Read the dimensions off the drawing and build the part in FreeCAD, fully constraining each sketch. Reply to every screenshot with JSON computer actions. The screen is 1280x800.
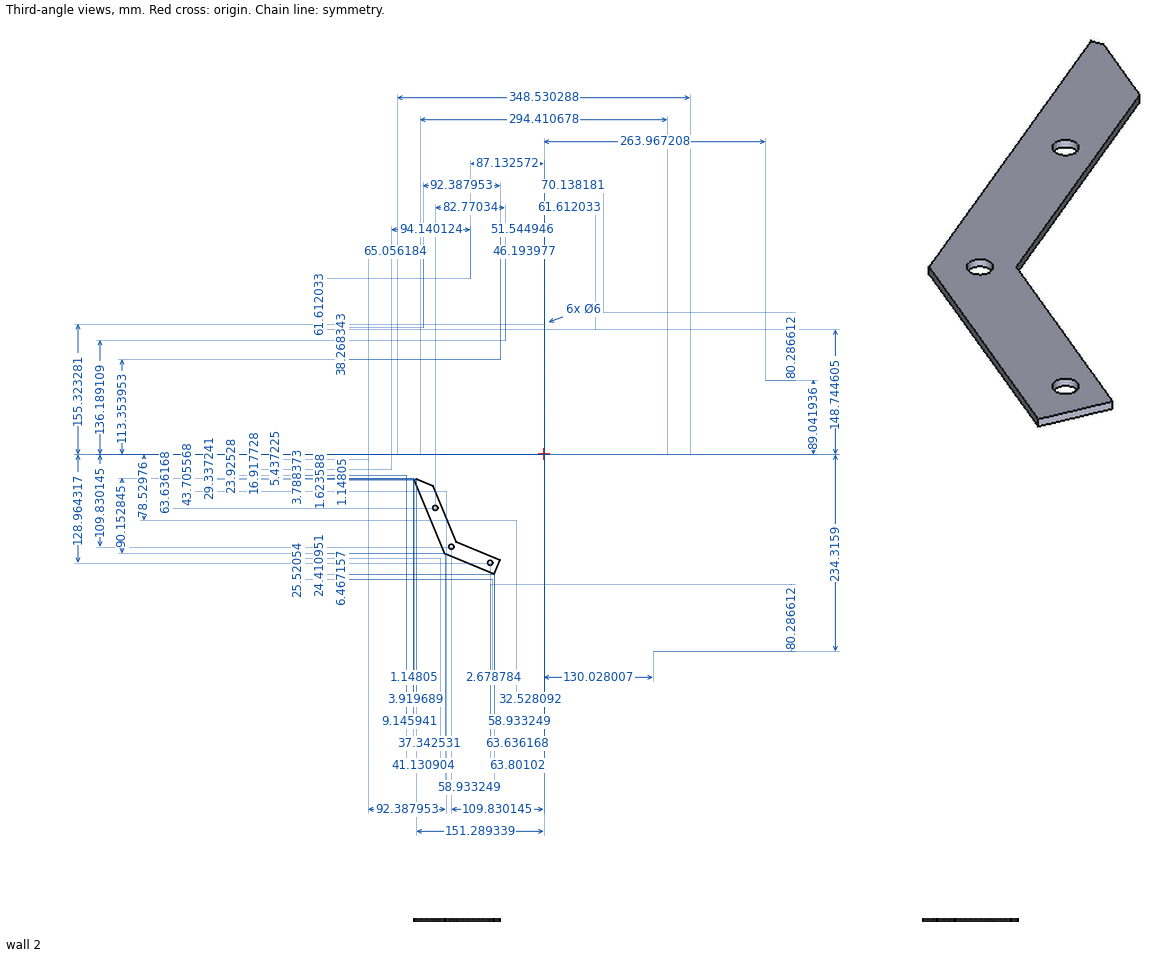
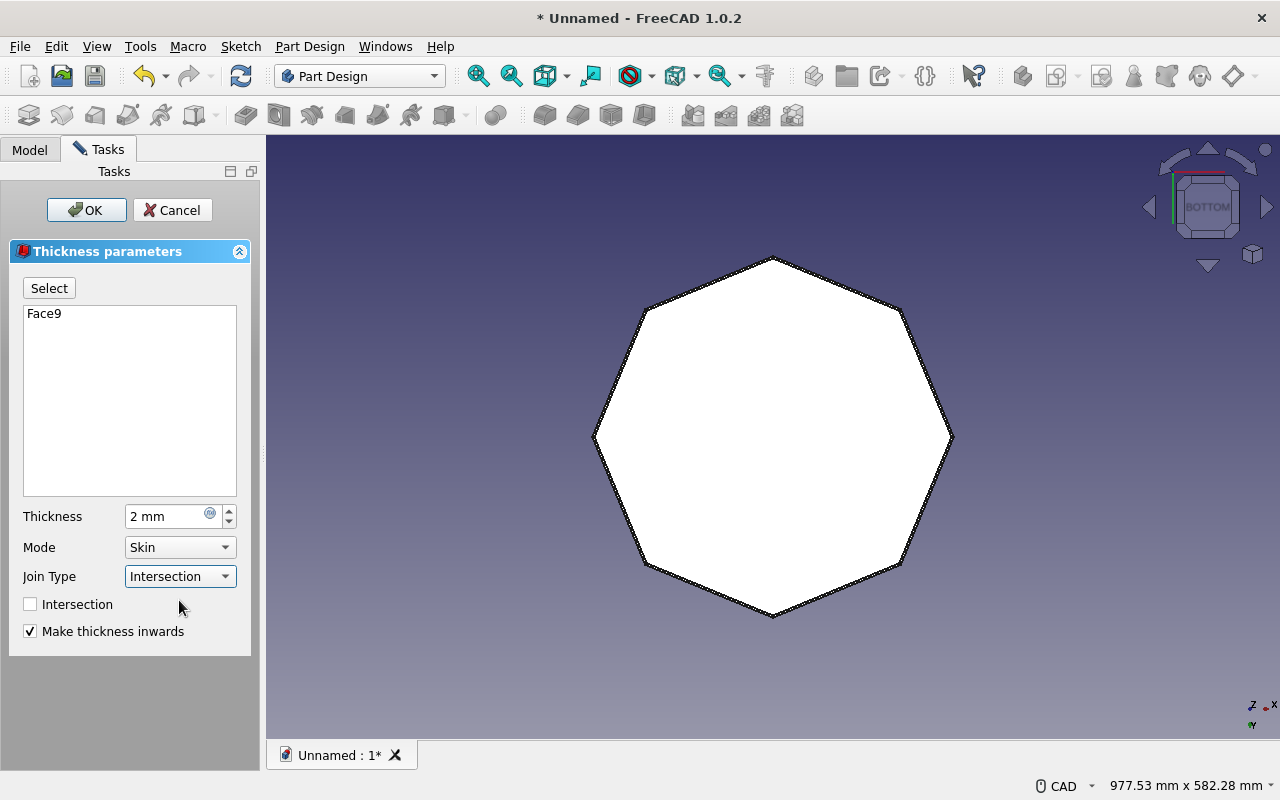
{"action": "left_click", "coordinate": [87, 210]}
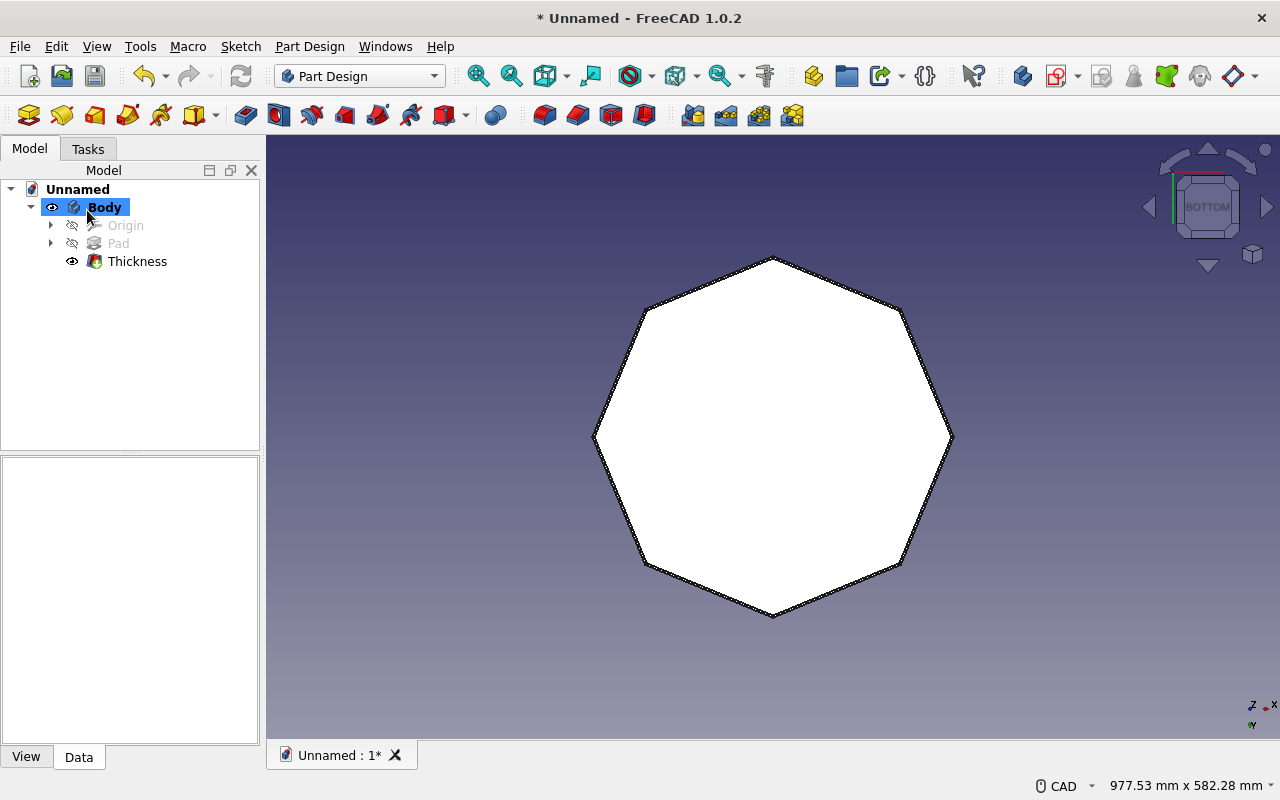
{"action": "key", "text": "0"}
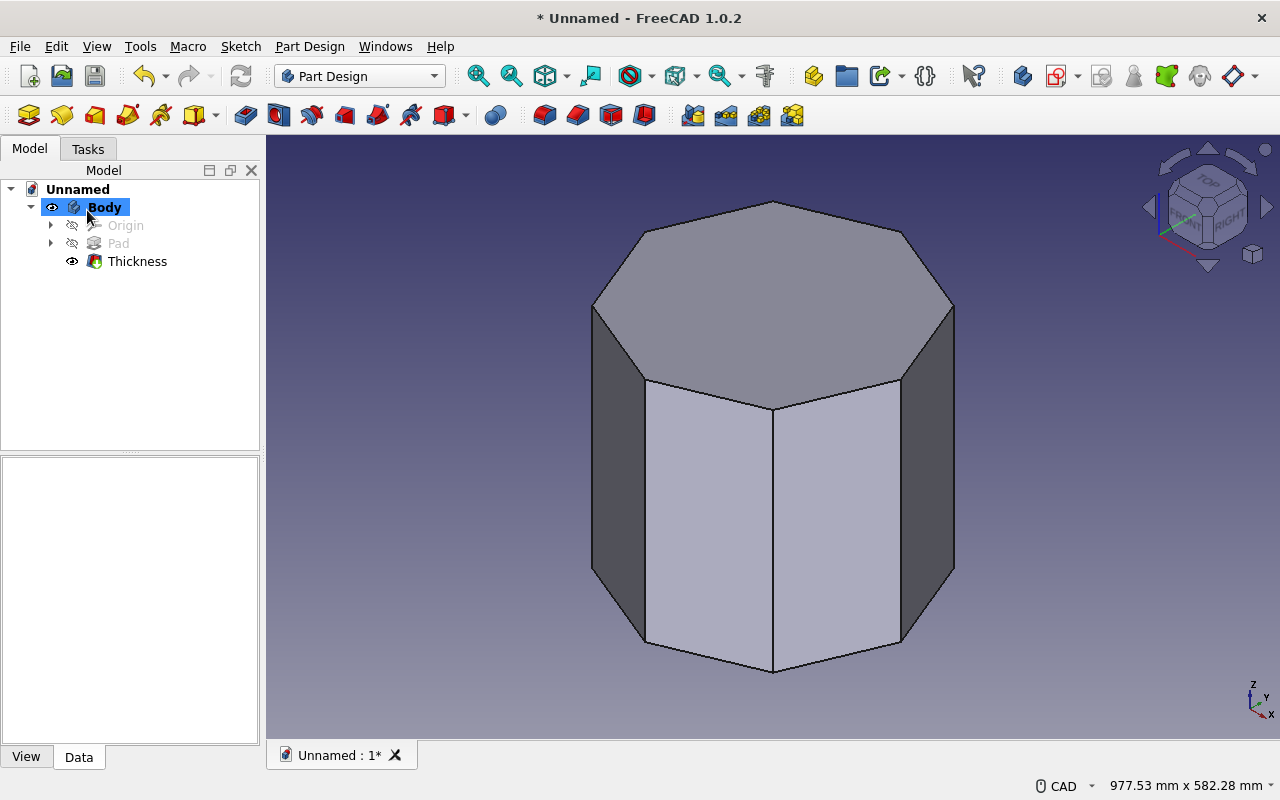
{"action": "left_click", "coordinate": [773, 305]}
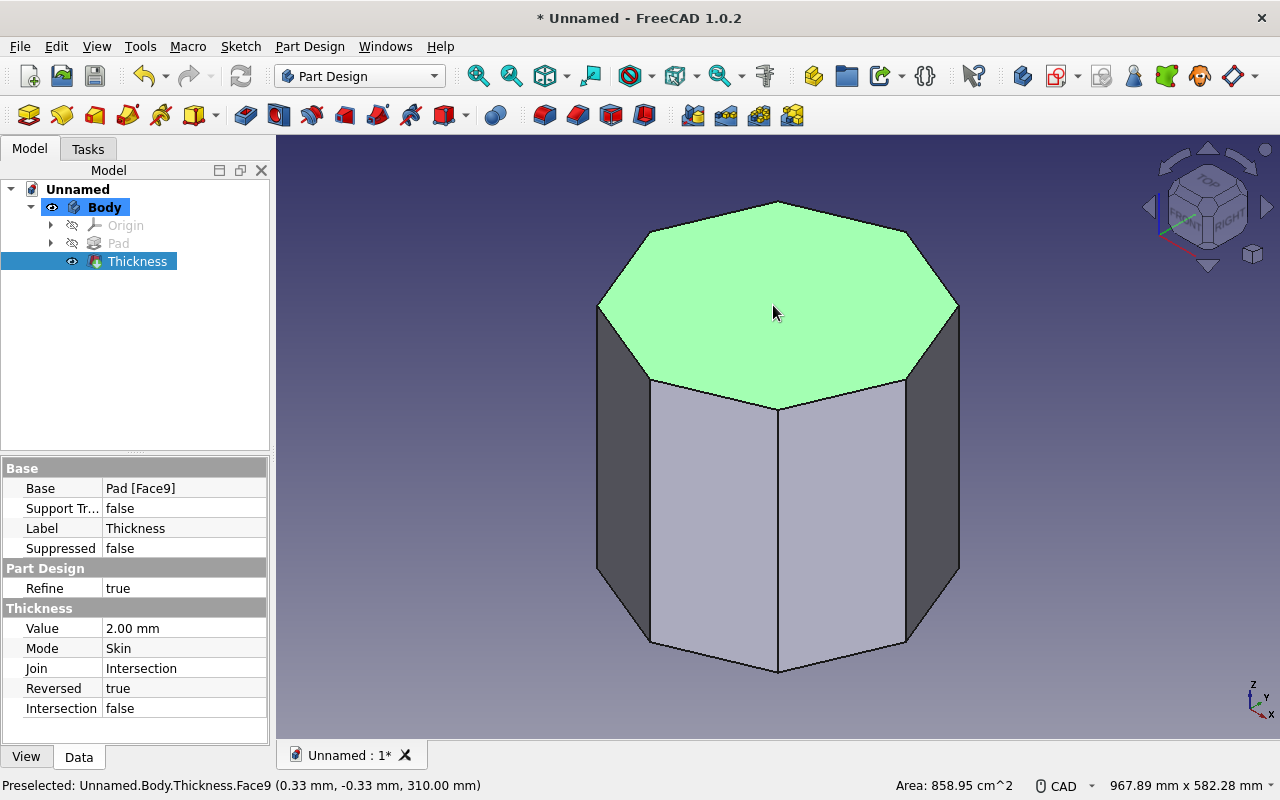
{"action": "left_click", "coordinate": [1056, 76]}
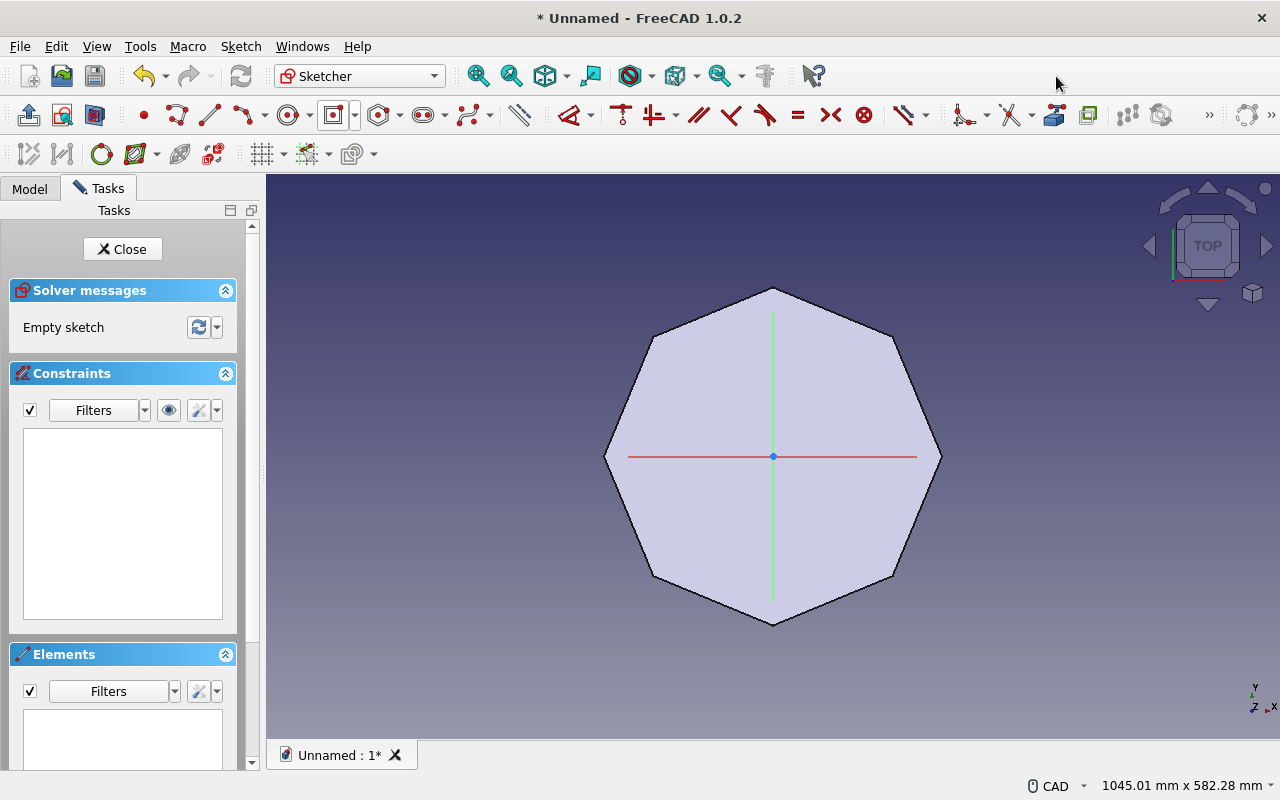
{"action": "left_click", "coordinate": [400, 116]}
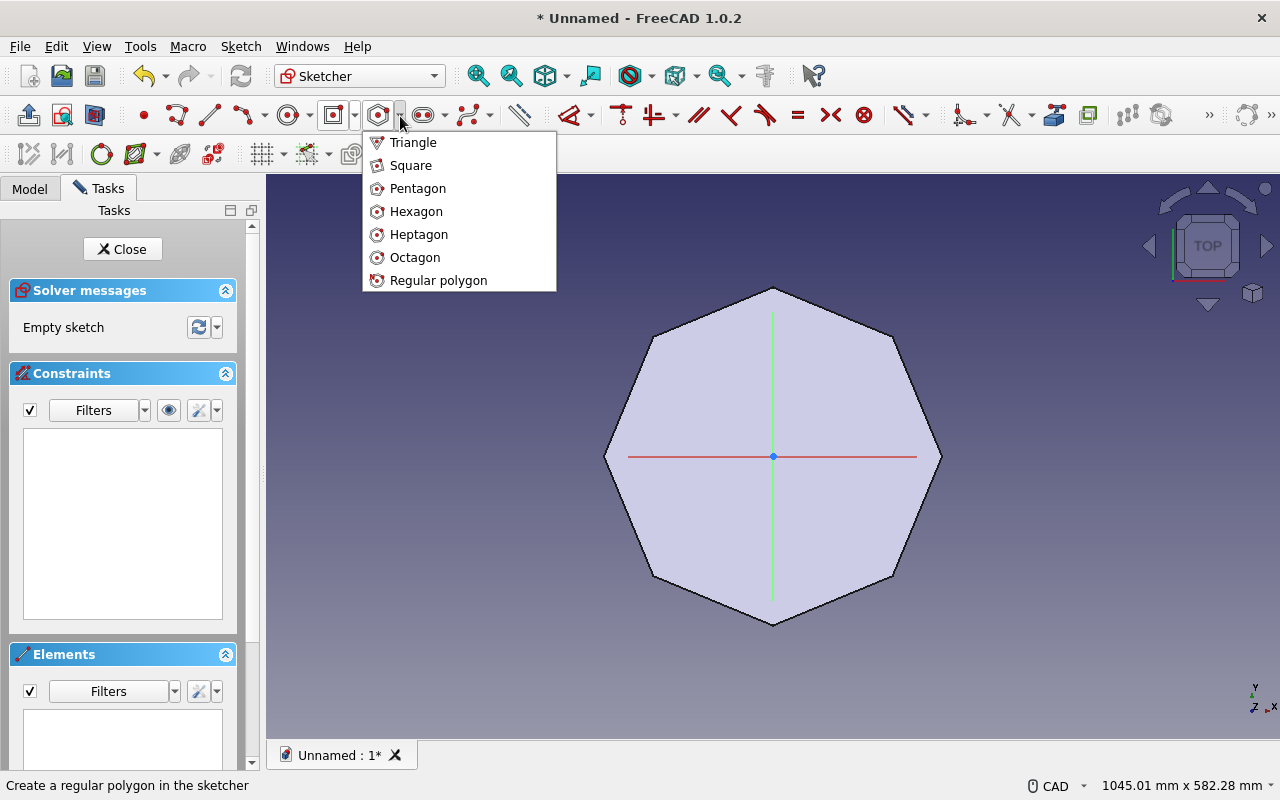
{"action": "left_click", "coordinate": [460, 258]}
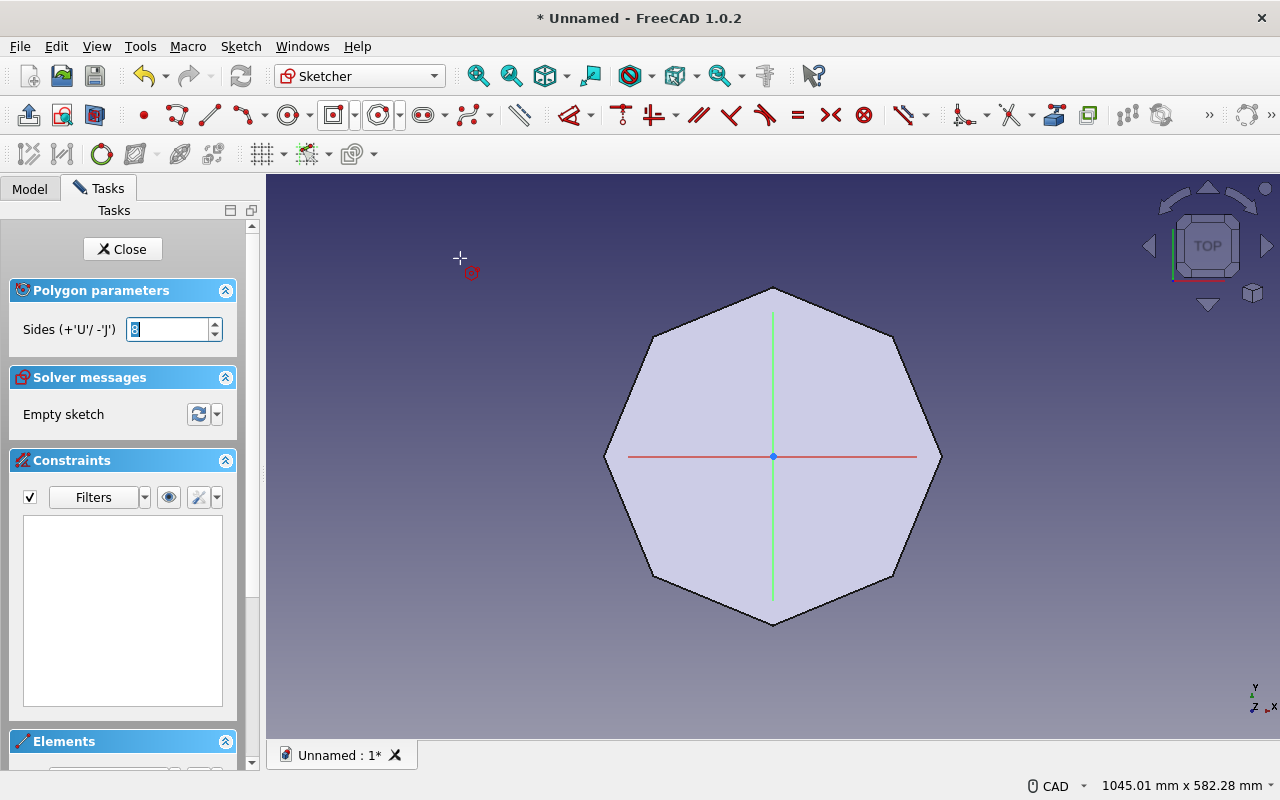
{"action": "left_click", "coordinate": [773, 456]}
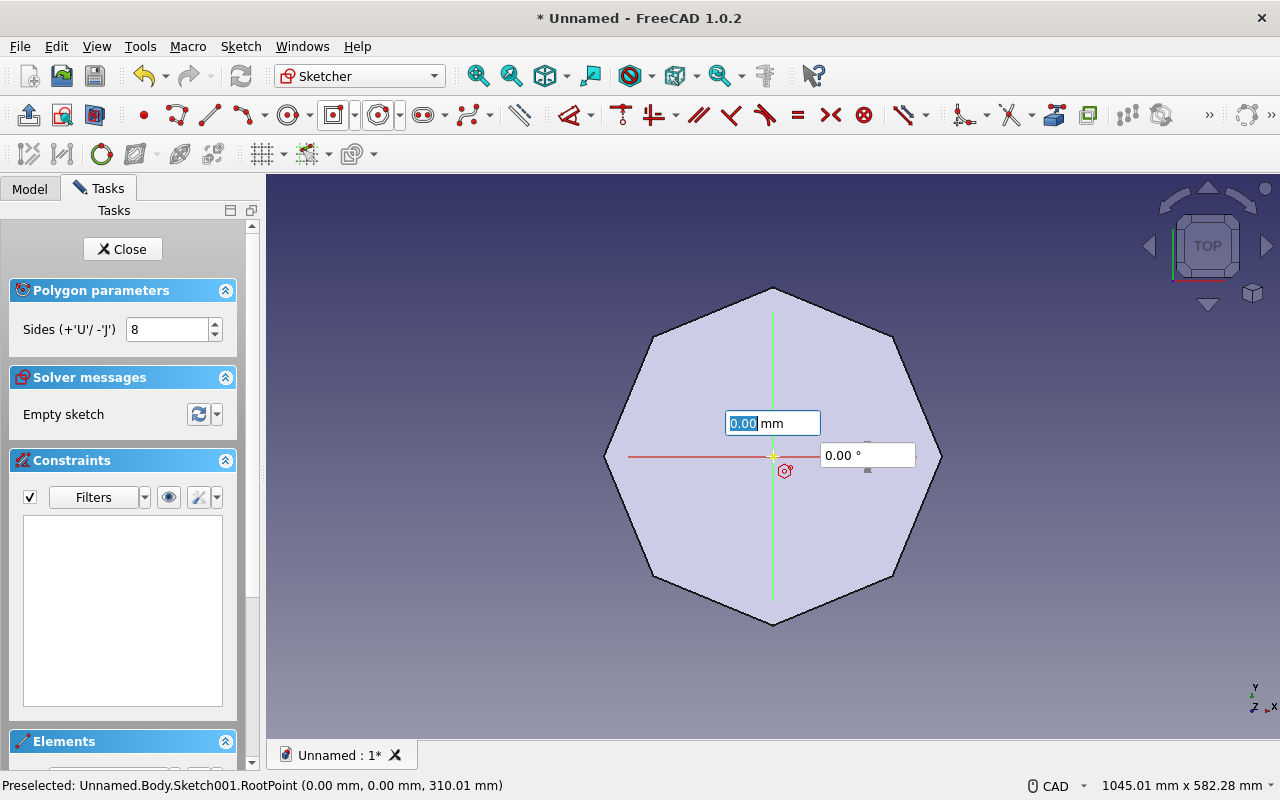
{"action": "left_click", "coordinate": [773, 314]}
{"action": "right_click", "coordinate": [773, 314]}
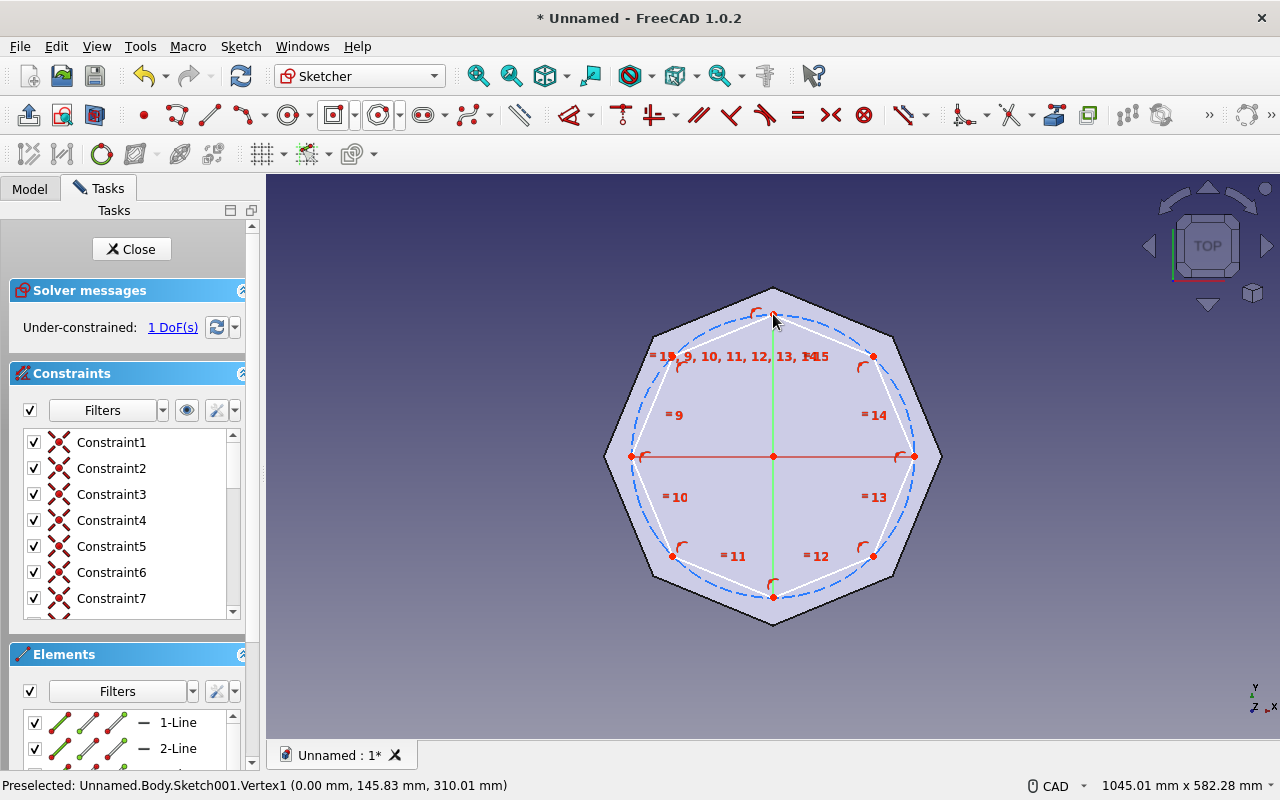
{"action": "left_click", "coordinate": [568, 116]}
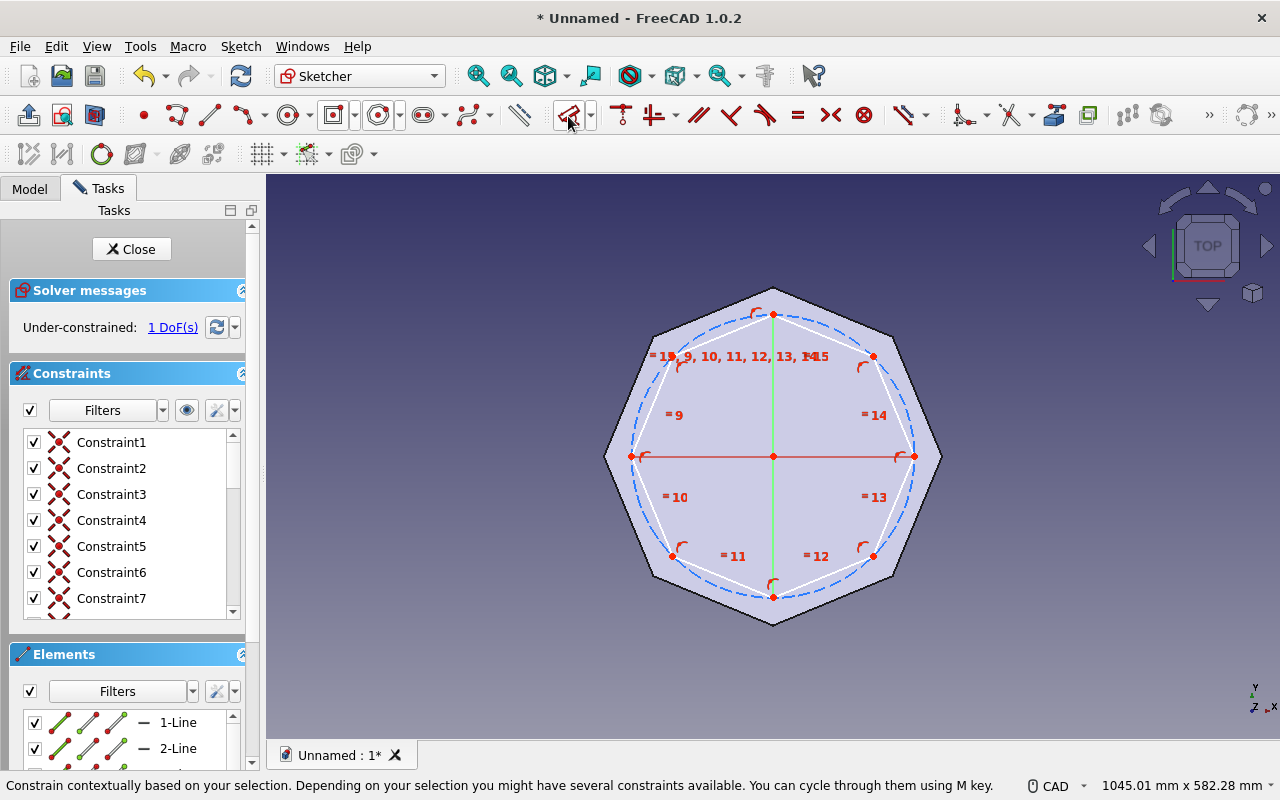
{"action": "left_click", "coordinate": [632, 456]}